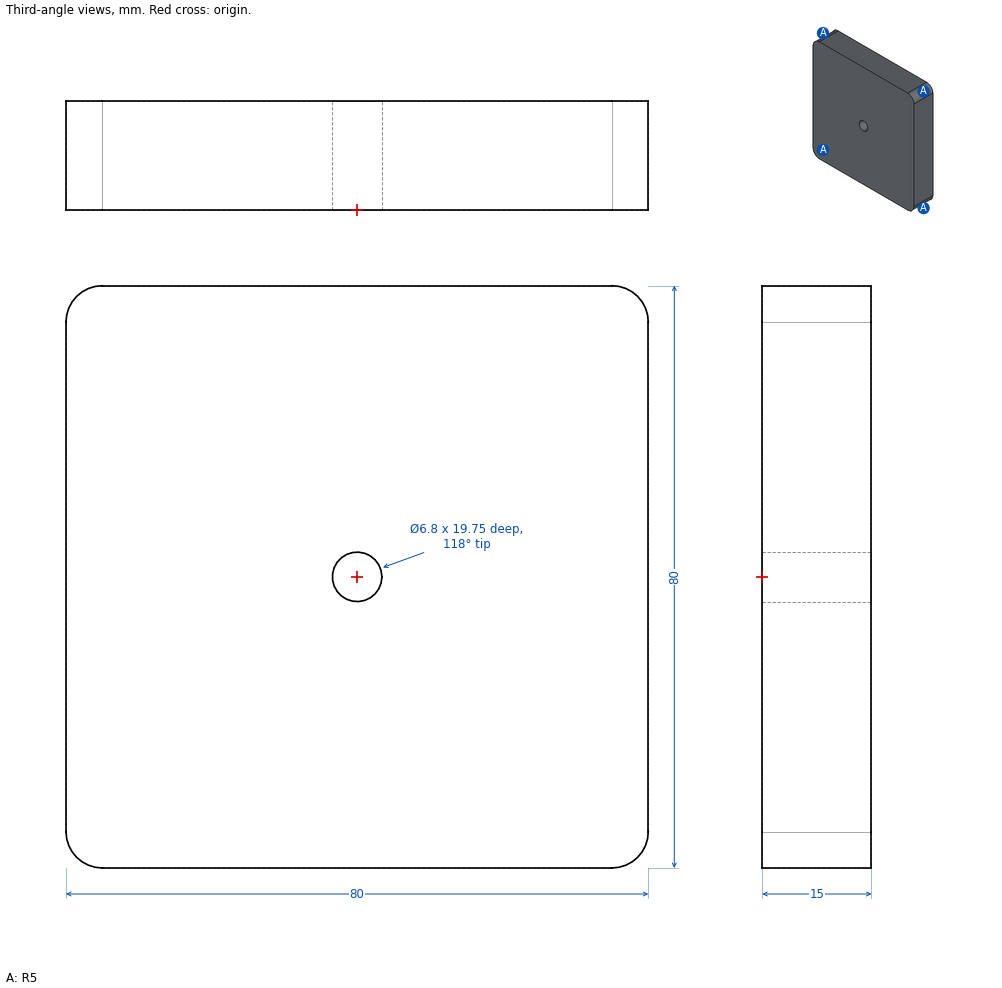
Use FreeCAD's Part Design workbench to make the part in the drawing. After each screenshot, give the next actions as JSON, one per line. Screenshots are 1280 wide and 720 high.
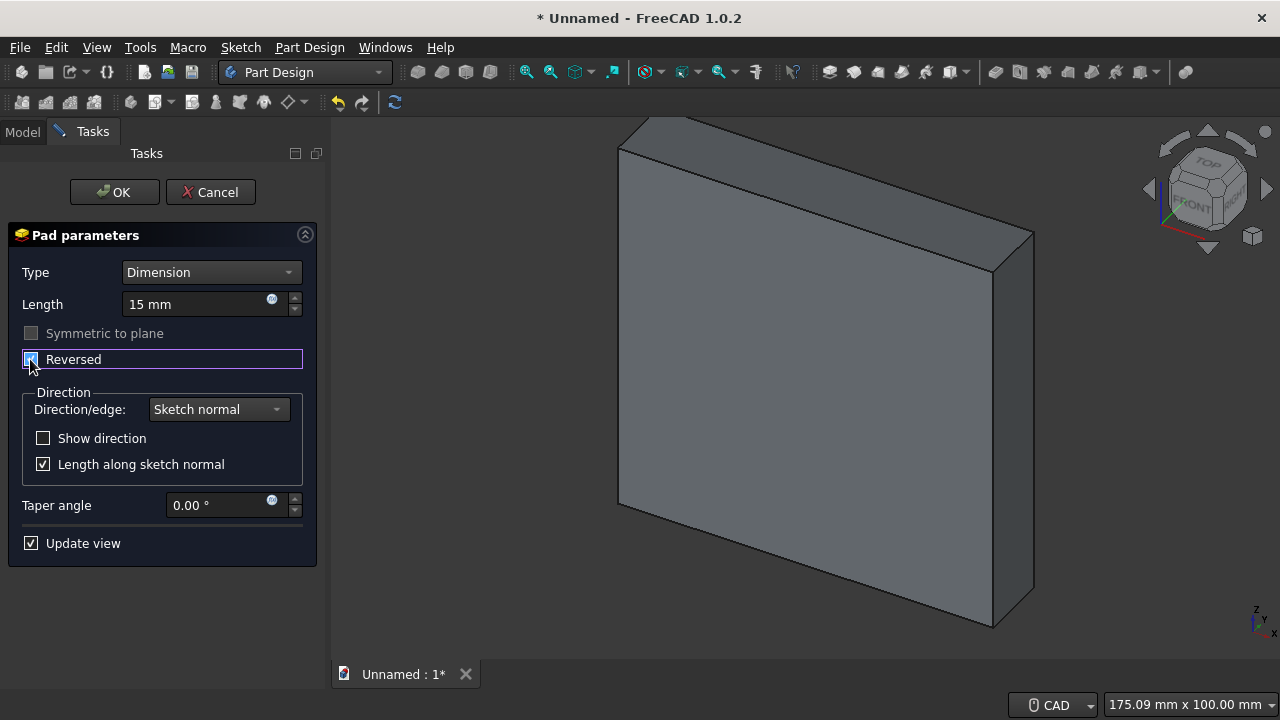
{"action": "left_click", "coordinate": [115, 192]}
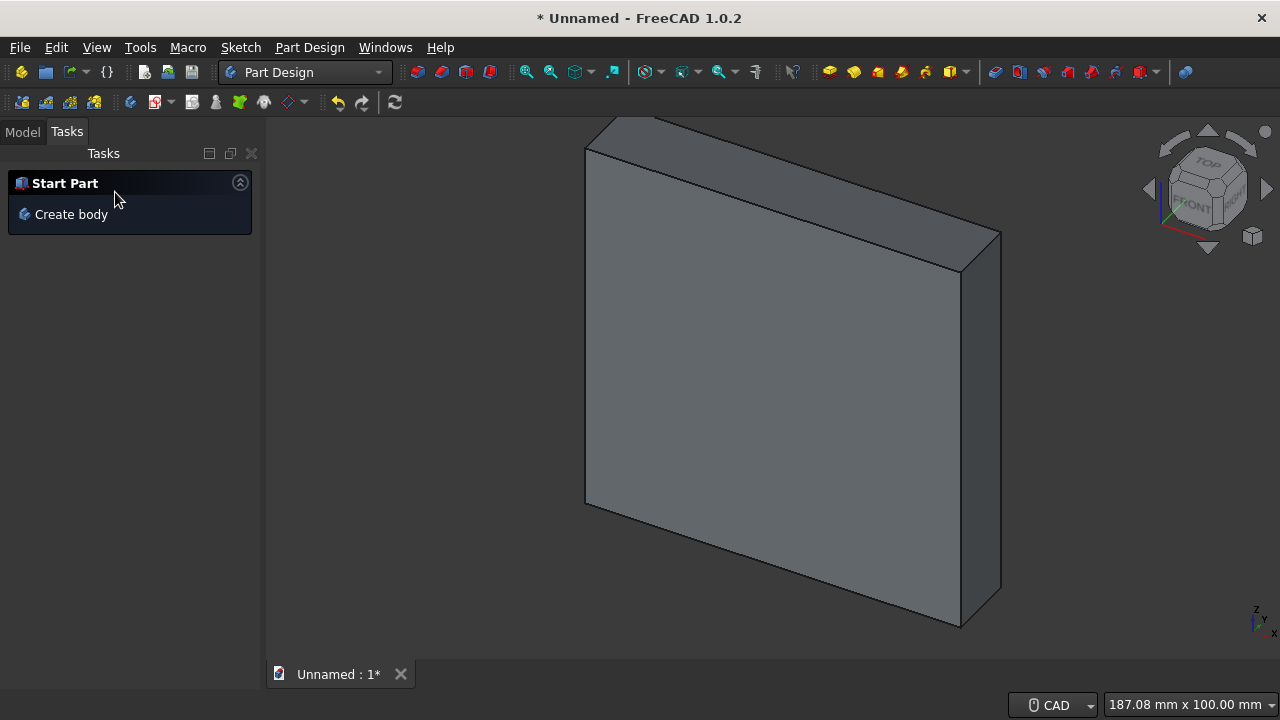
{"action": "left_click", "coordinate": [528, 72]}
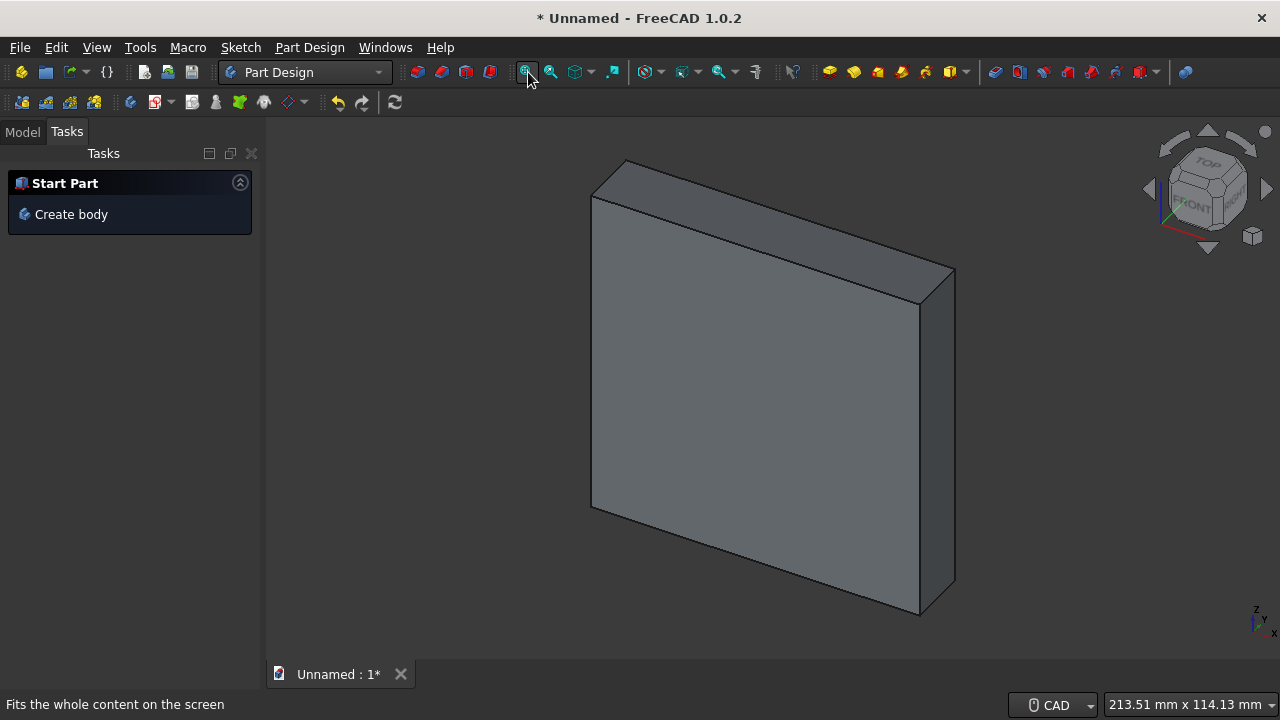
{"action": "left_click", "coordinate": [938, 286]}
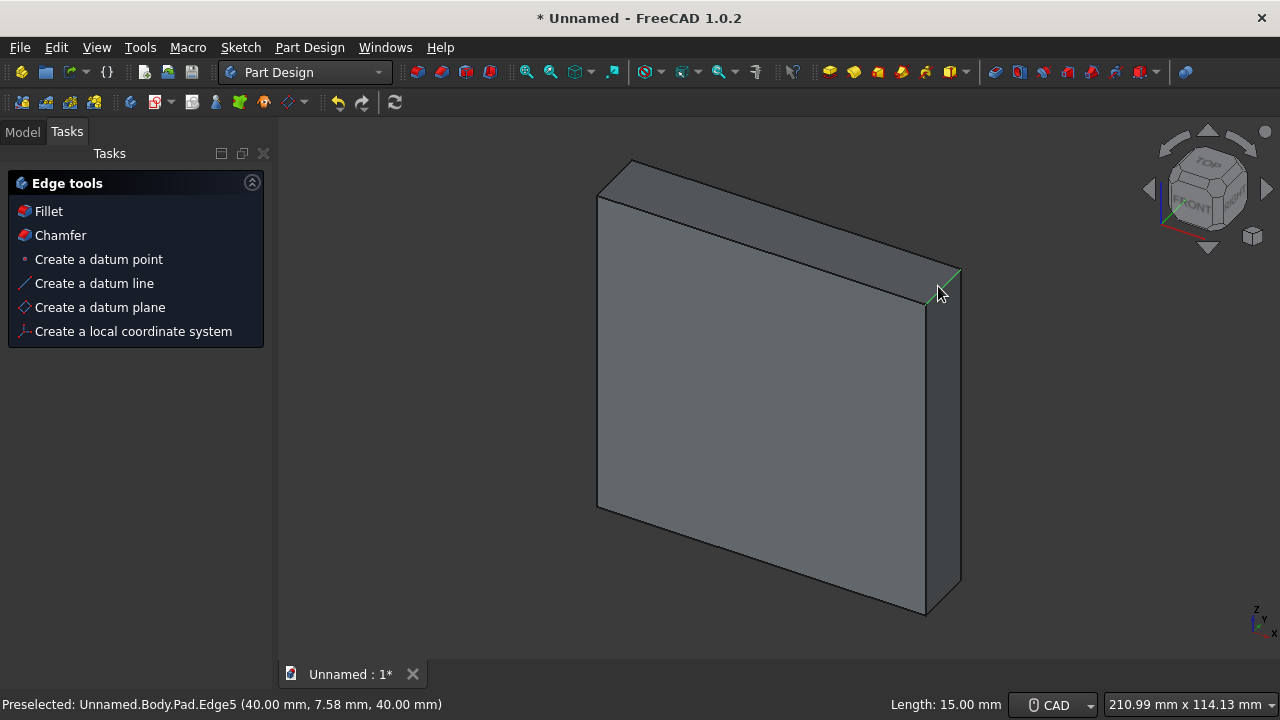
{"action": "key", "text": "0"}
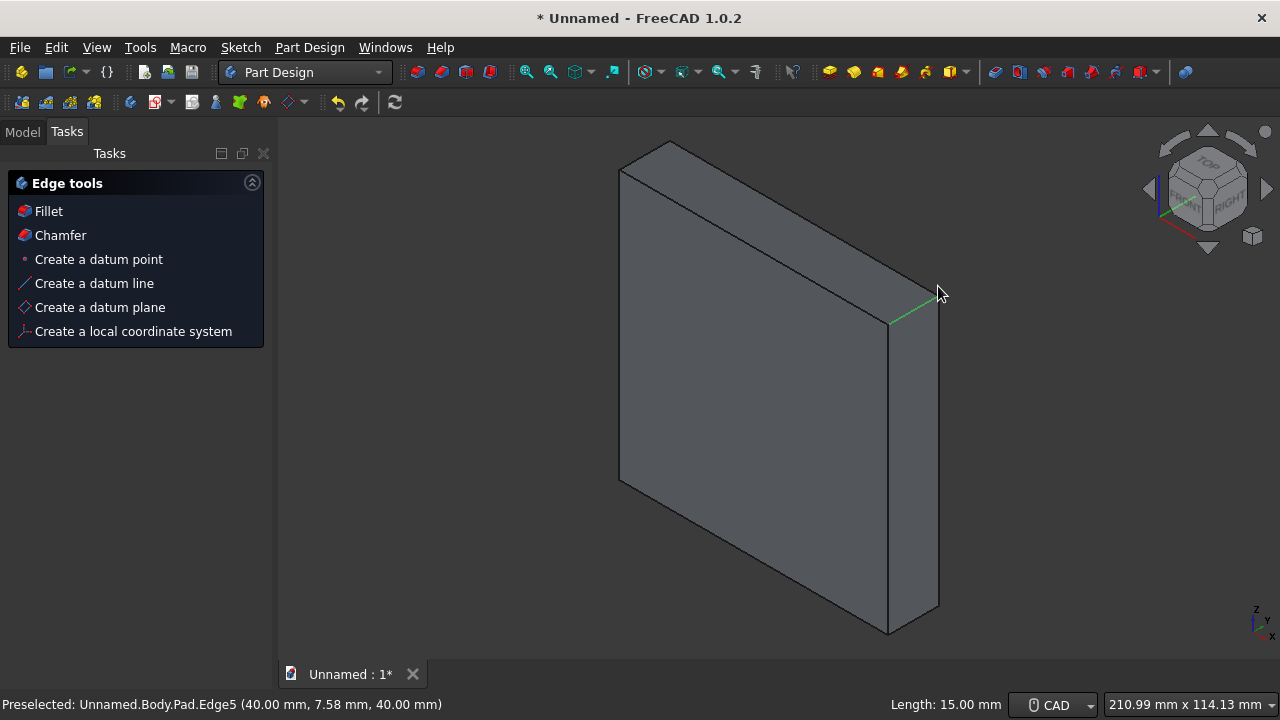
{"action": "key", "text": "2"}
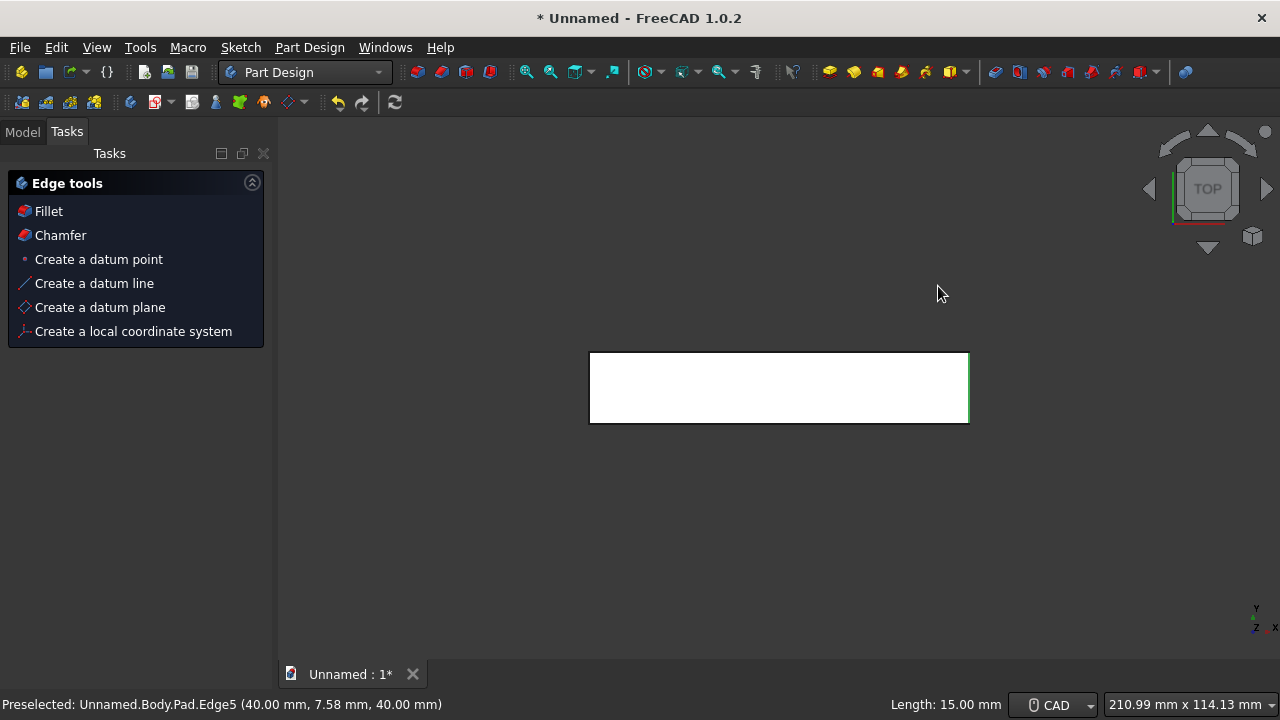
{"action": "key", "text": "v f"}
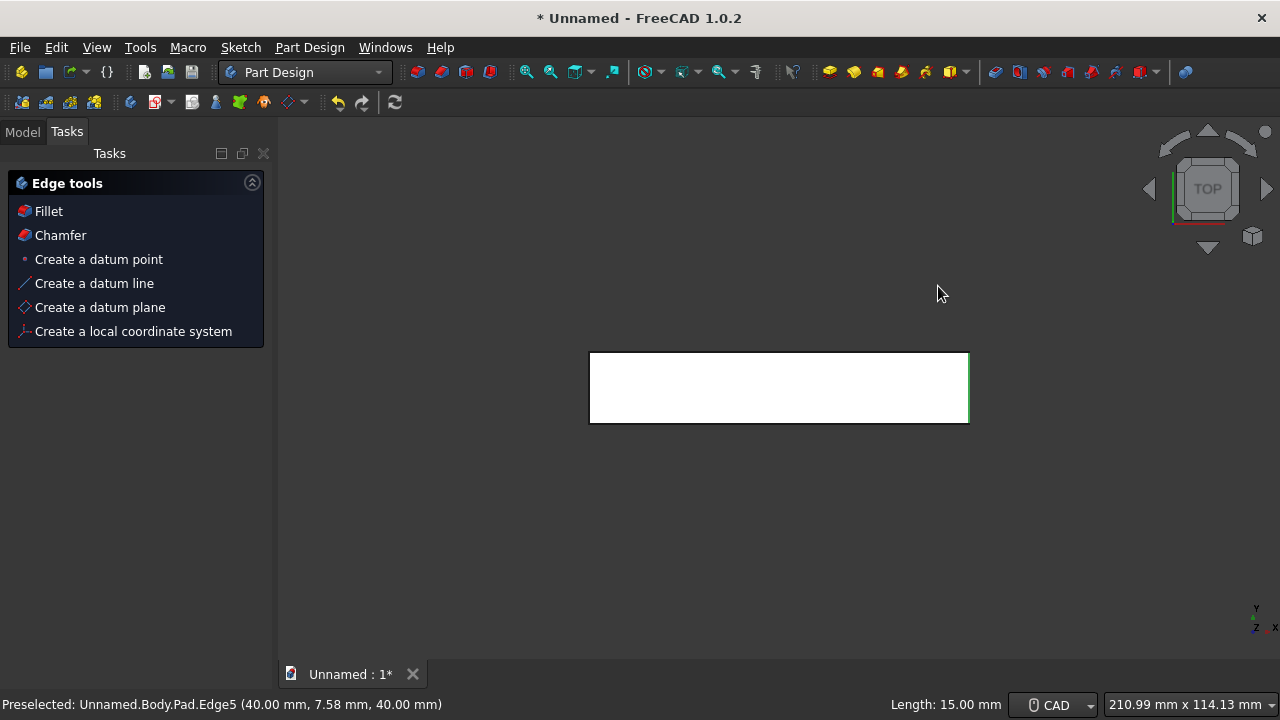
{"action": "left_click", "coordinate": [589, 387], "text": "ctrl"}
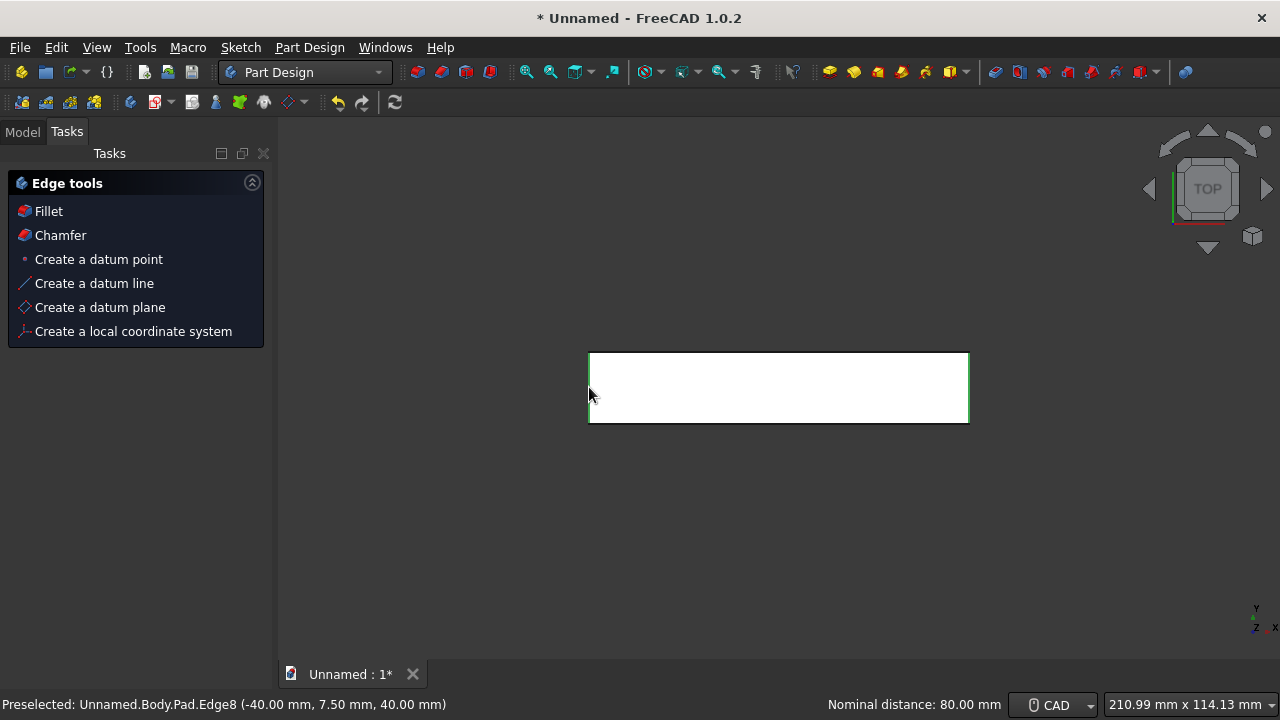
{"action": "key", "text": "1"}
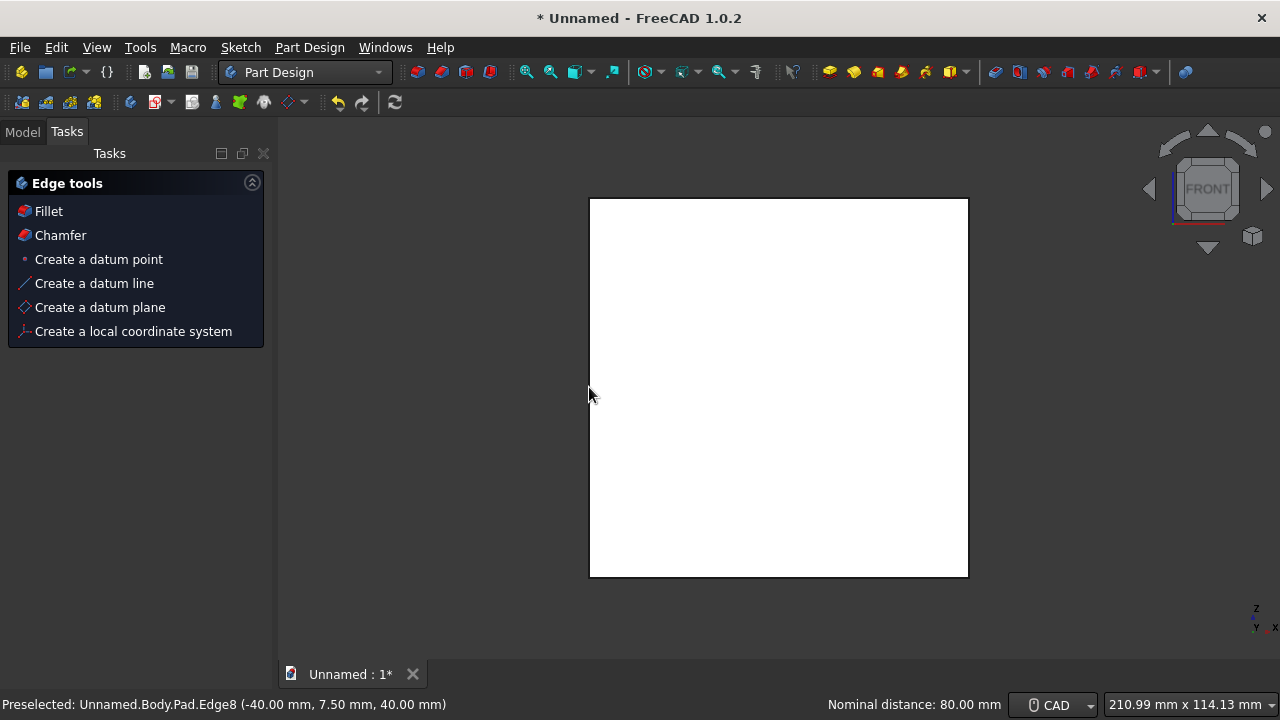
{"action": "key", "text": "3"}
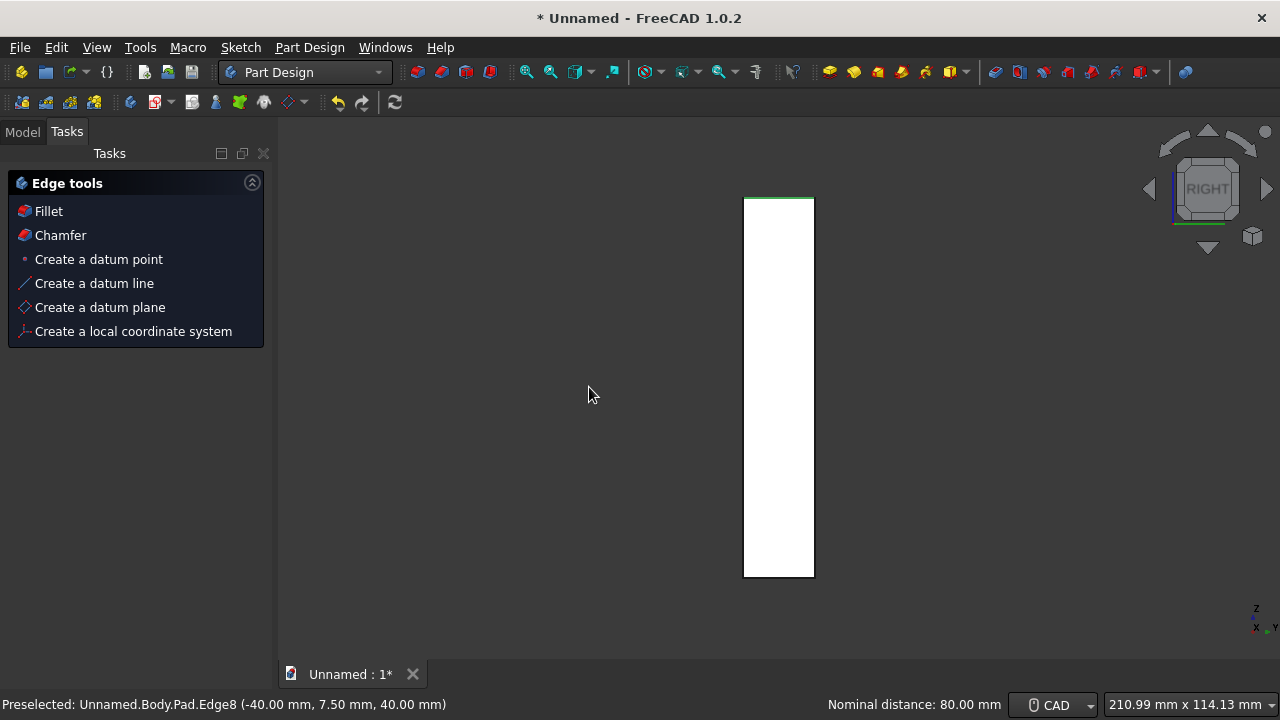
{"action": "left_click", "coordinate": [779, 577], "text": "ctrl"}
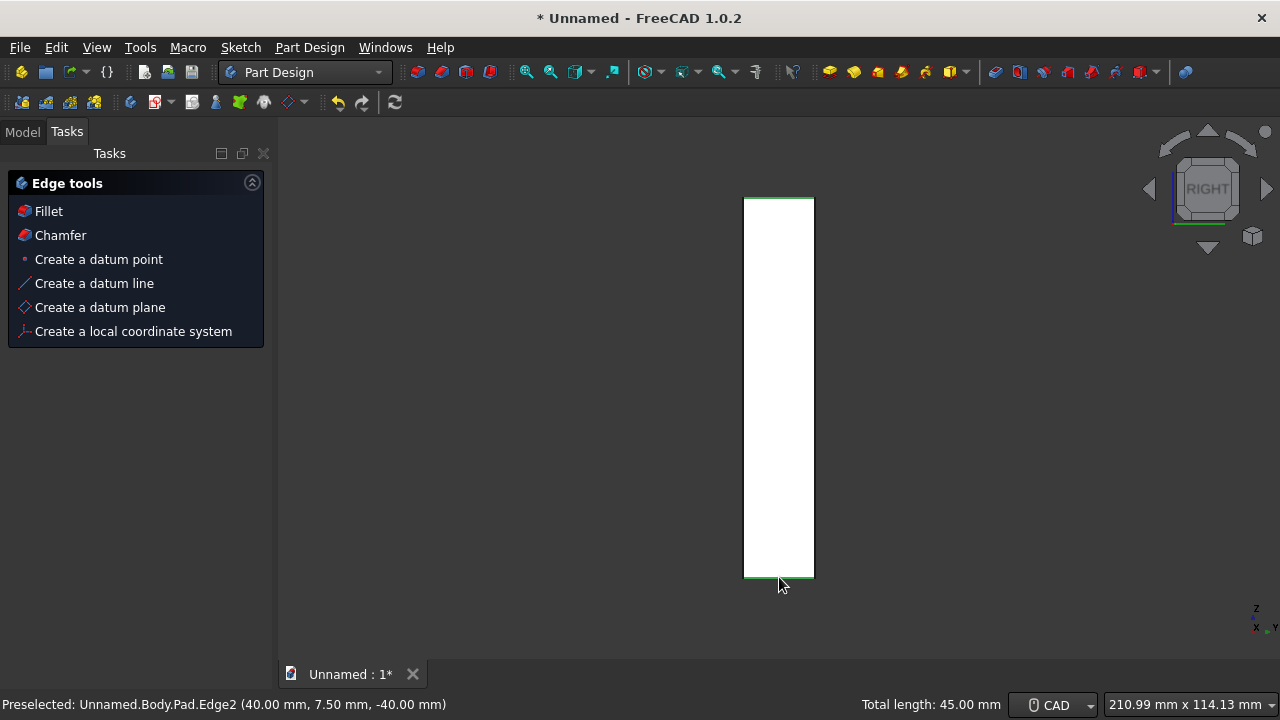
{"action": "key", "text": "5"}